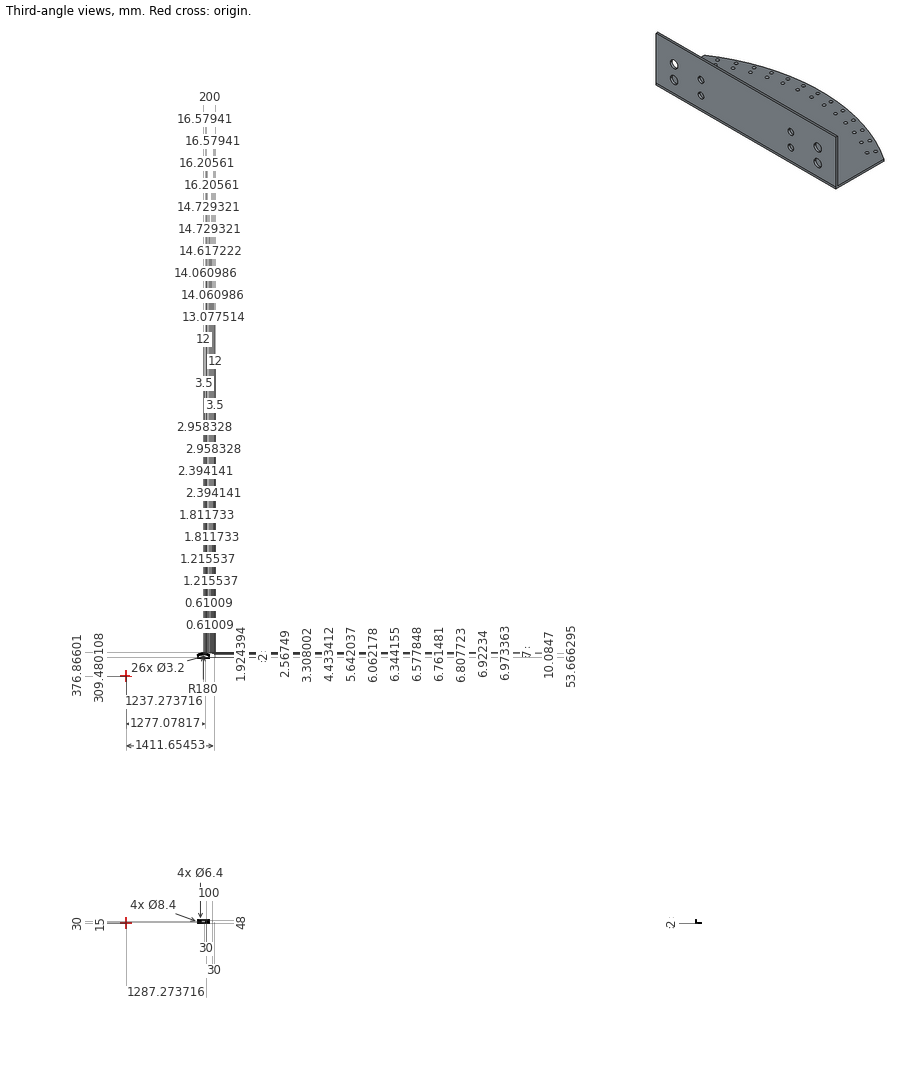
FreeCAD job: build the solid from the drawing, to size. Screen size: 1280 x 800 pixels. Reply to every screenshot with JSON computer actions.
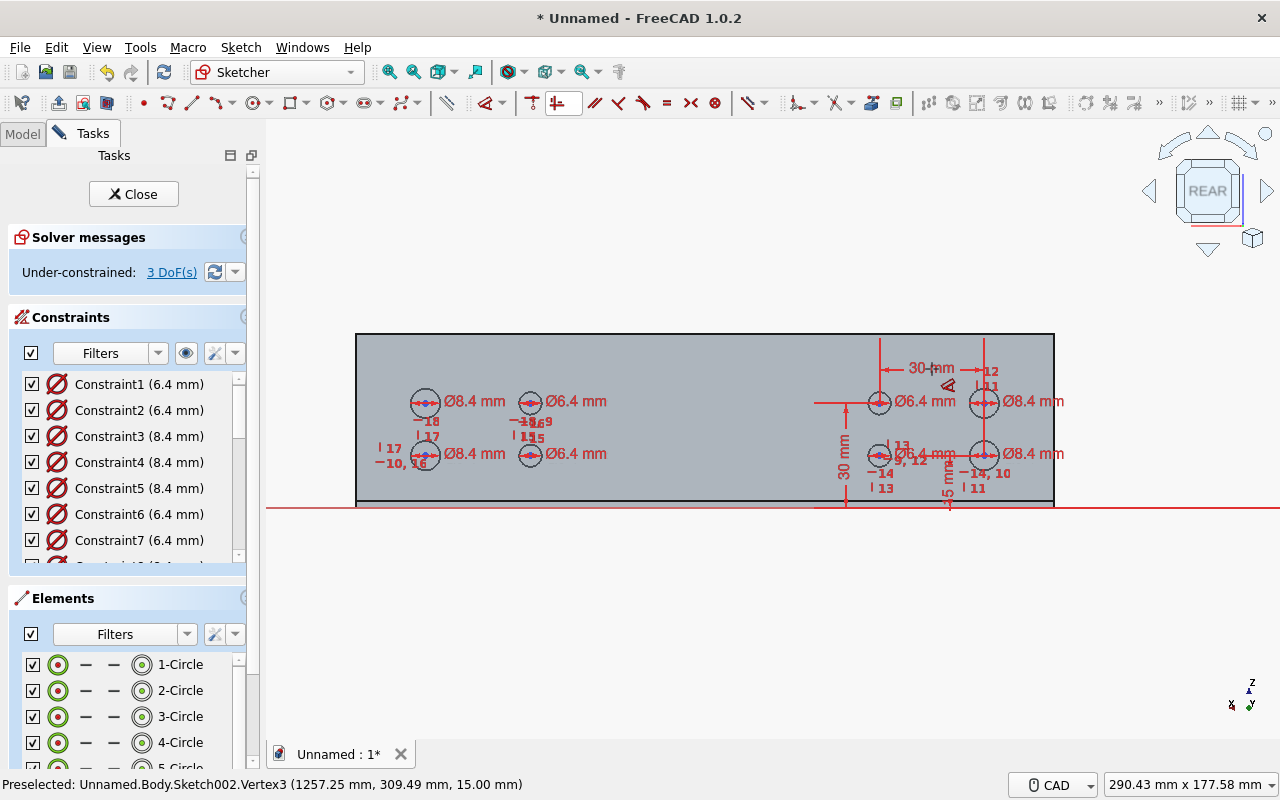
{"action": "left_click", "coordinate": [530, 403]}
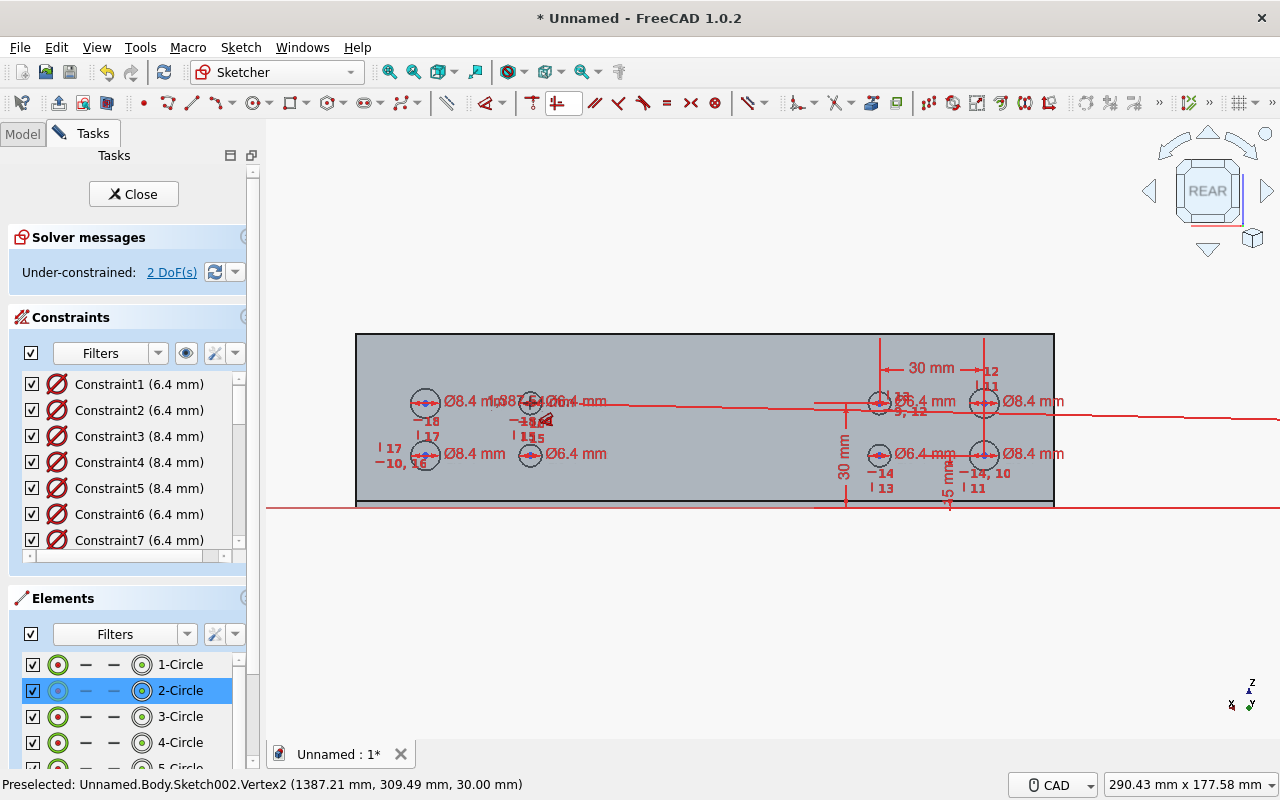
{"action": "left_click", "coordinate": [426, 456]}
{"action": "left_click", "coordinate": [478, 490]}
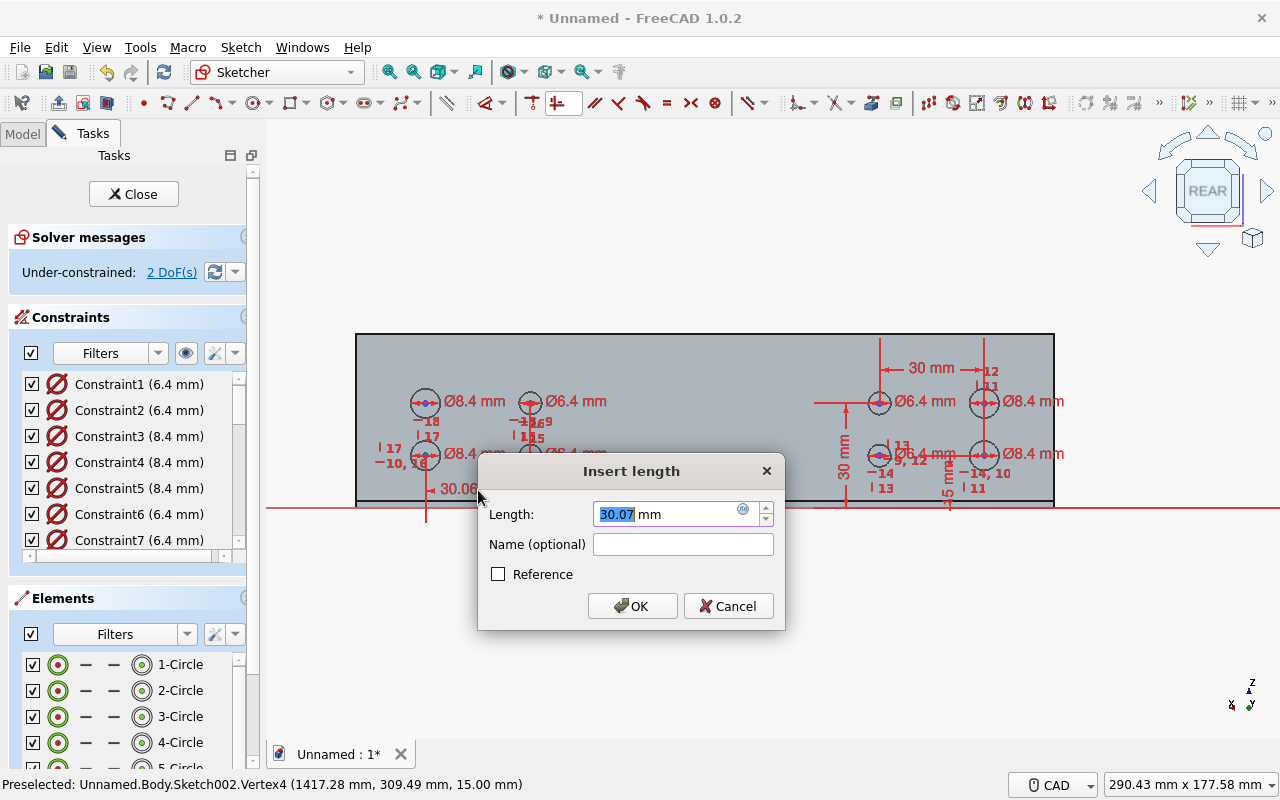
{"action": "type", "text": "30"}
{"action": "key", "text": "Return"}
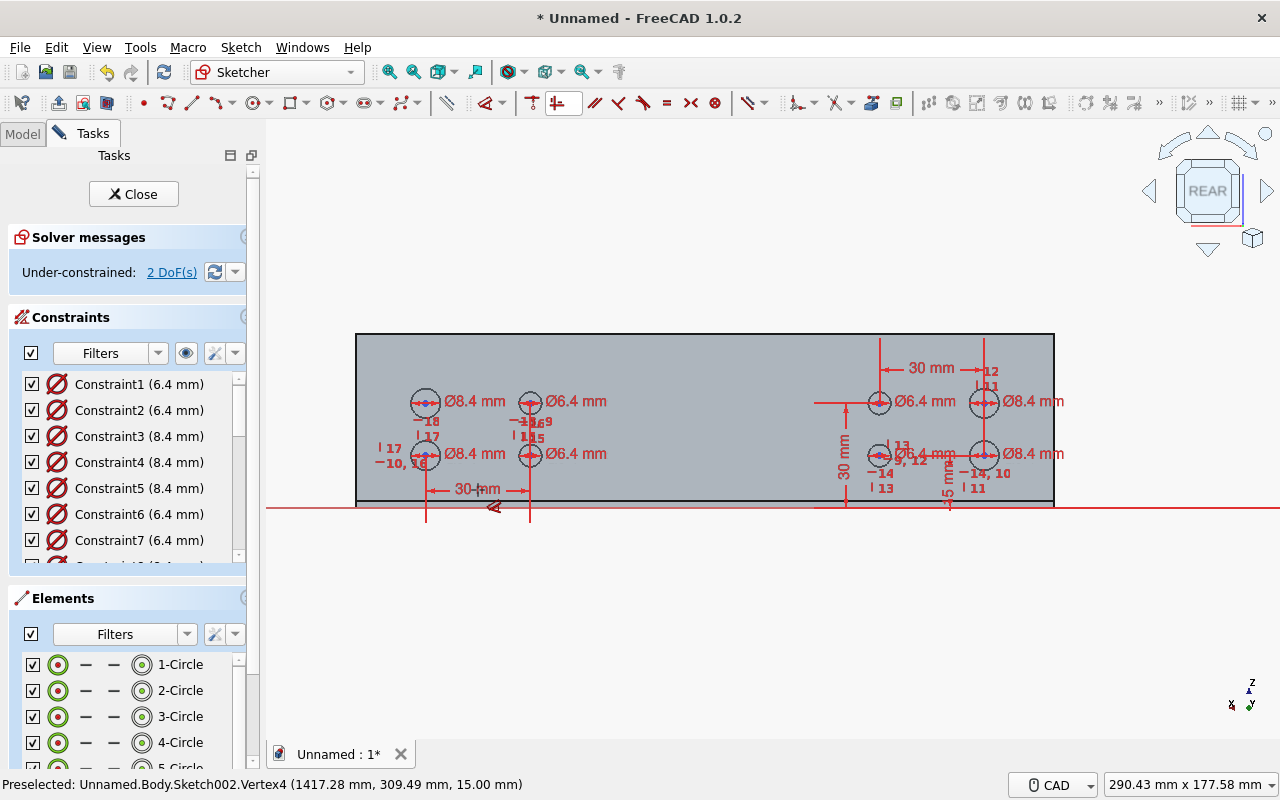
{"action": "left_click", "coordinate": [880, 403]}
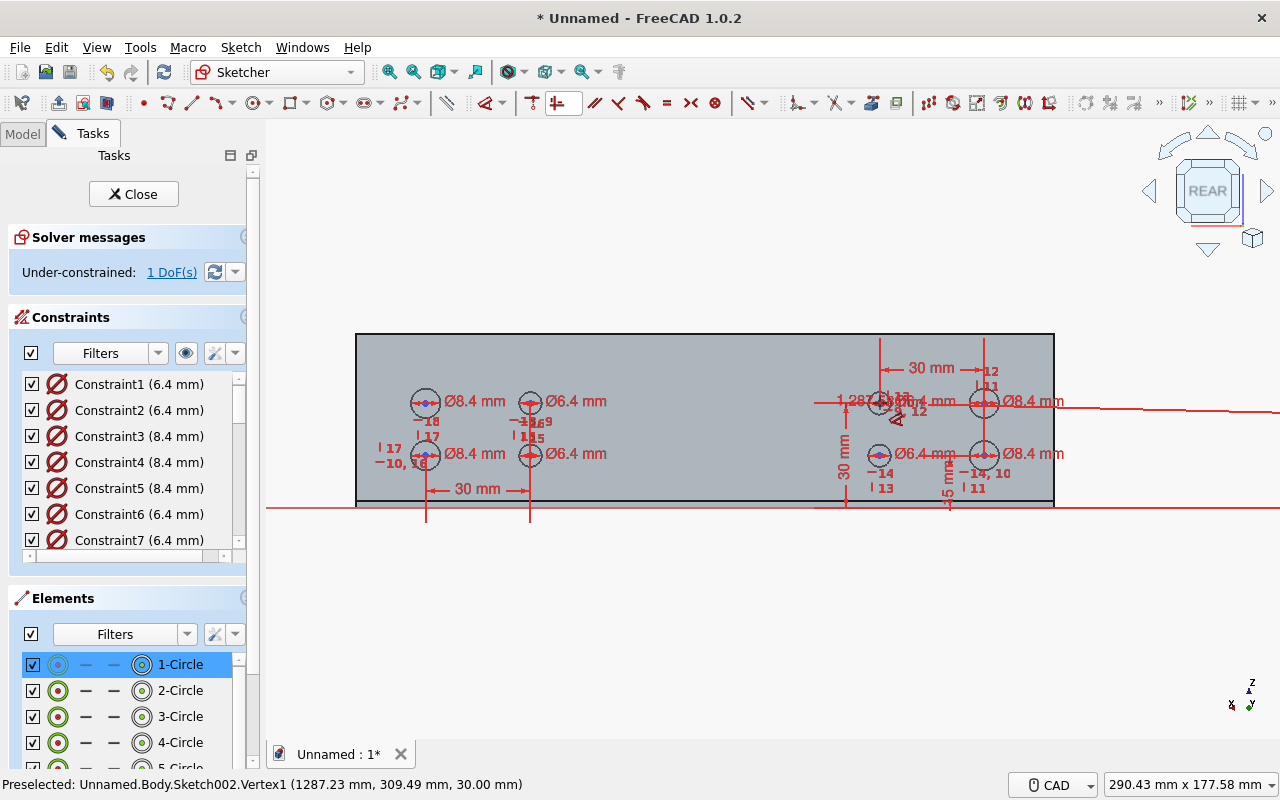
{"action": "left_click", "coordinate": [530, 403]}
{"action": "left_click", "coordinate": [705, 369]}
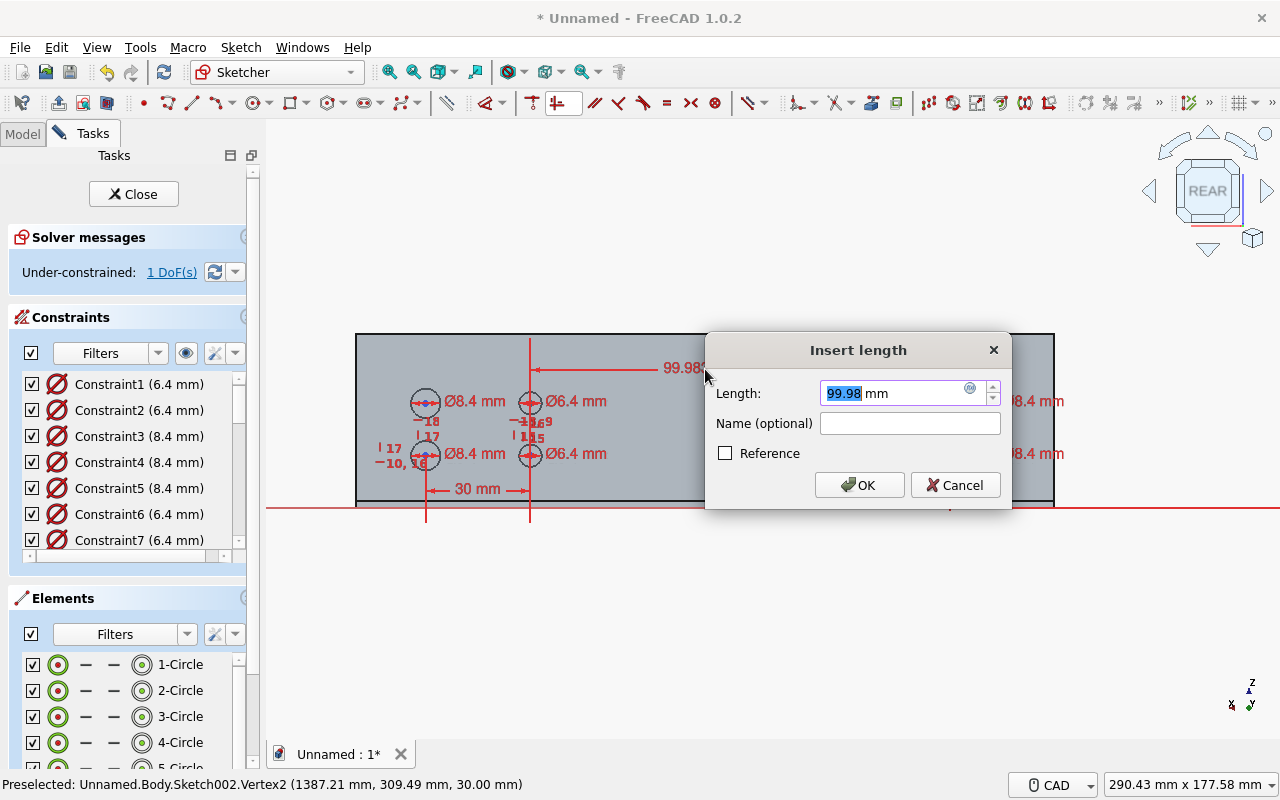
{"action": "type", "text": "100"}
{"action": "key", "text": "Return"}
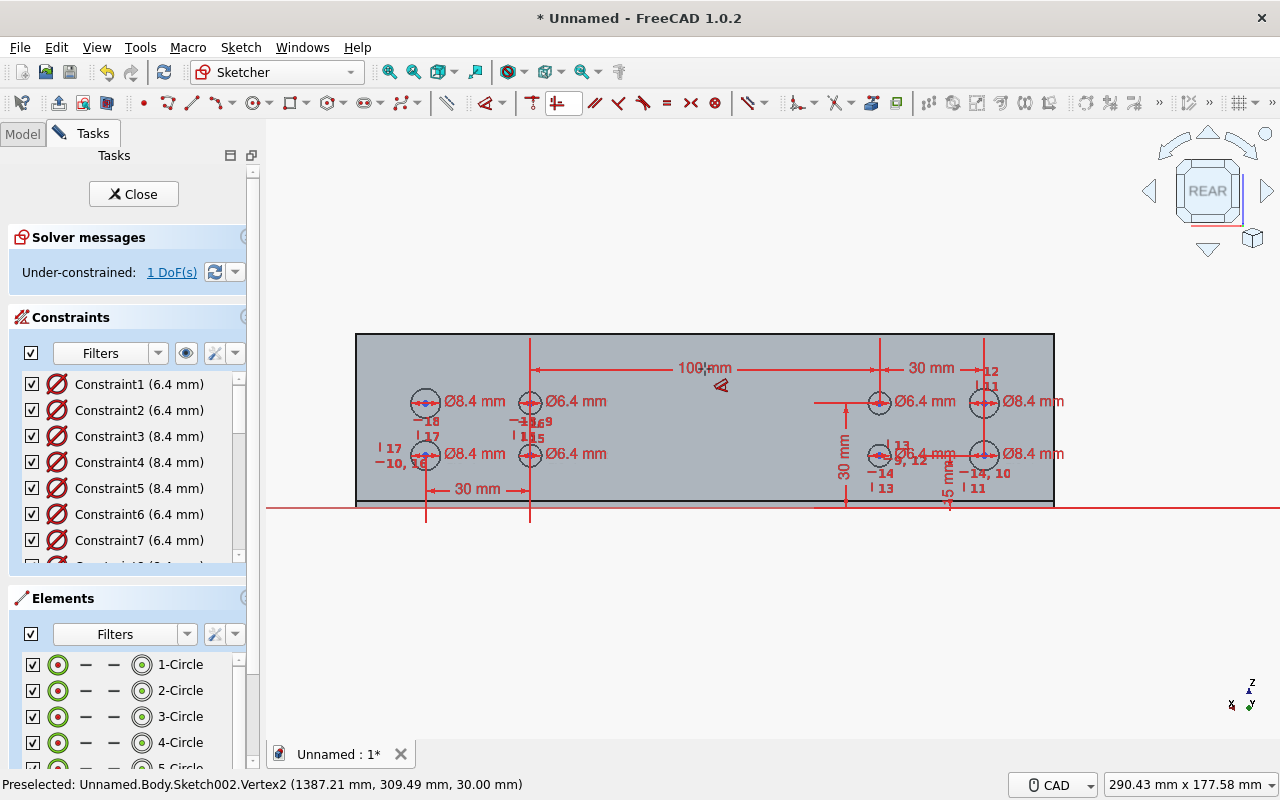
{"action": "left_click", "coordinate": [880, 403]}
{"action": "left_click", "coordinate": [997, 542]}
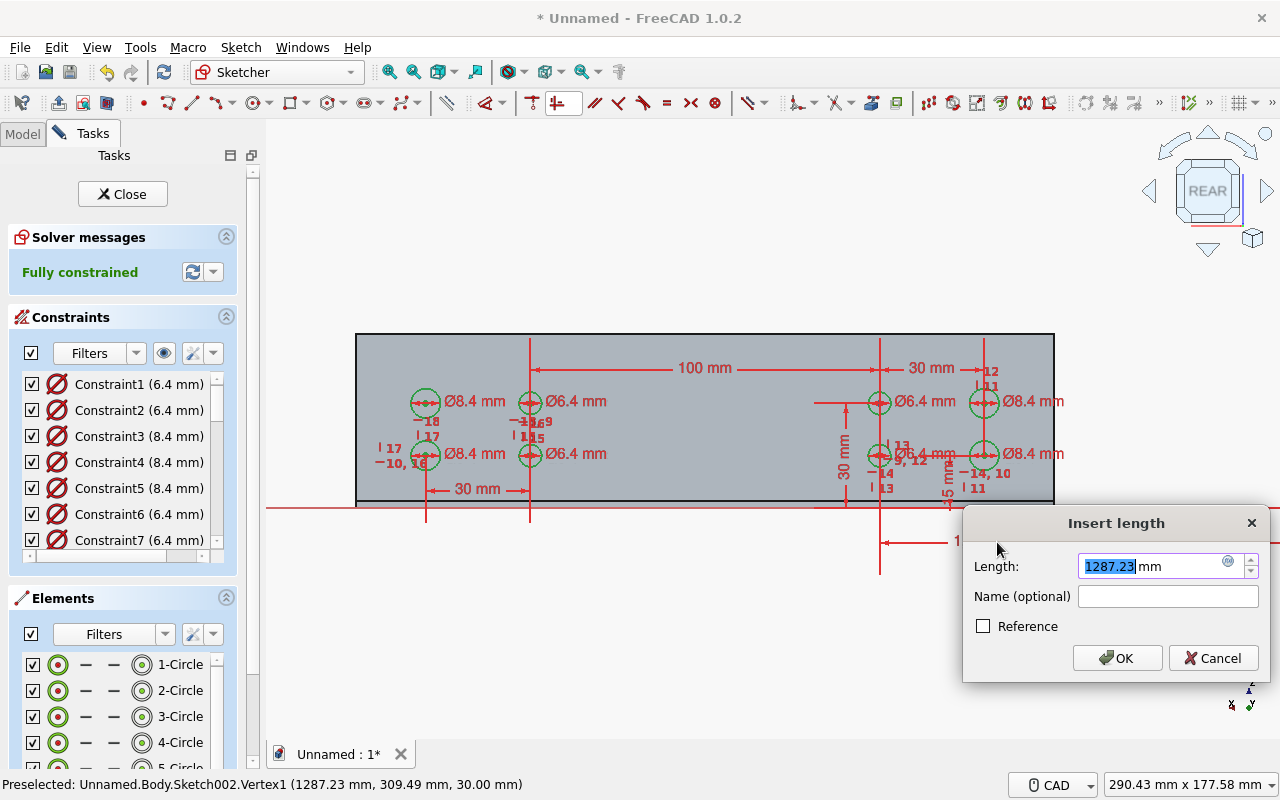
{"action": "type", "text": "1287.273716"}
{"action": "key", "text": "Return"}
{"action": "key", "text": "Escape"}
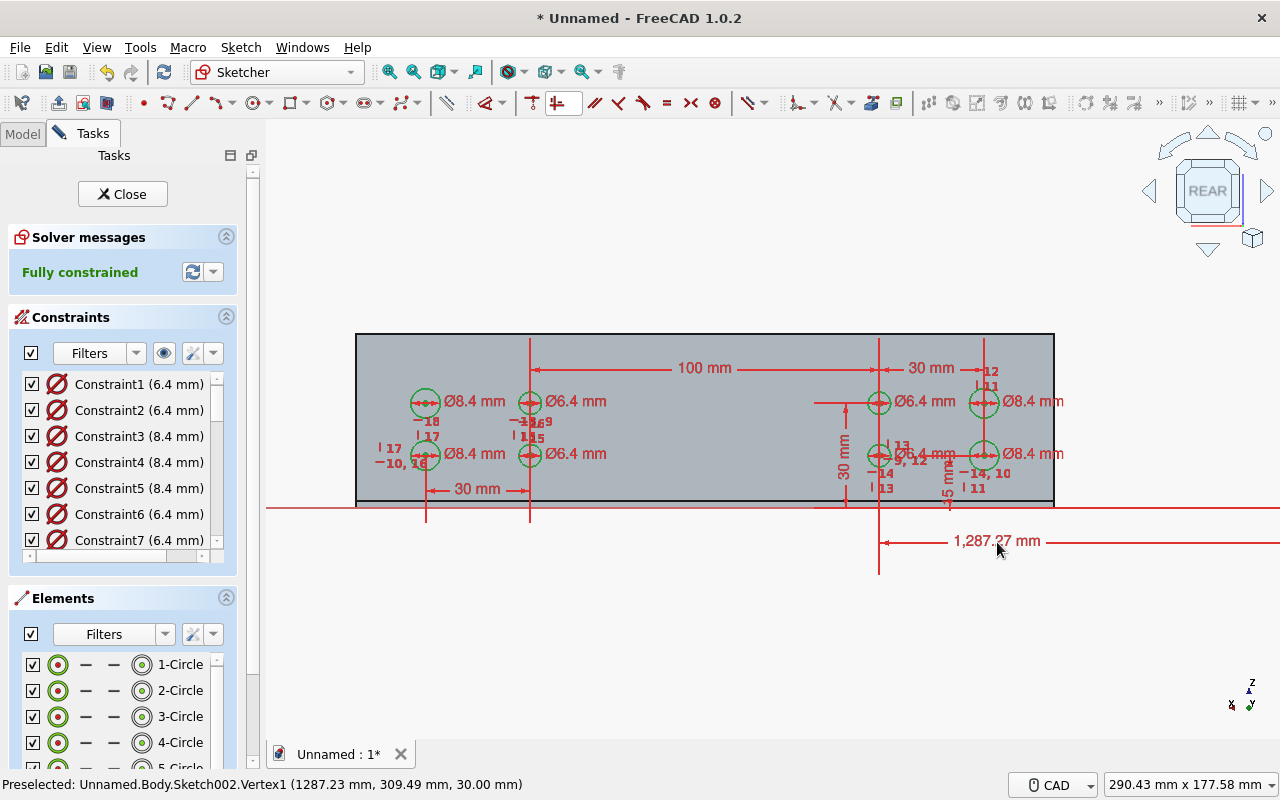
{"action": "left_click", "coordinate": [123, 194]}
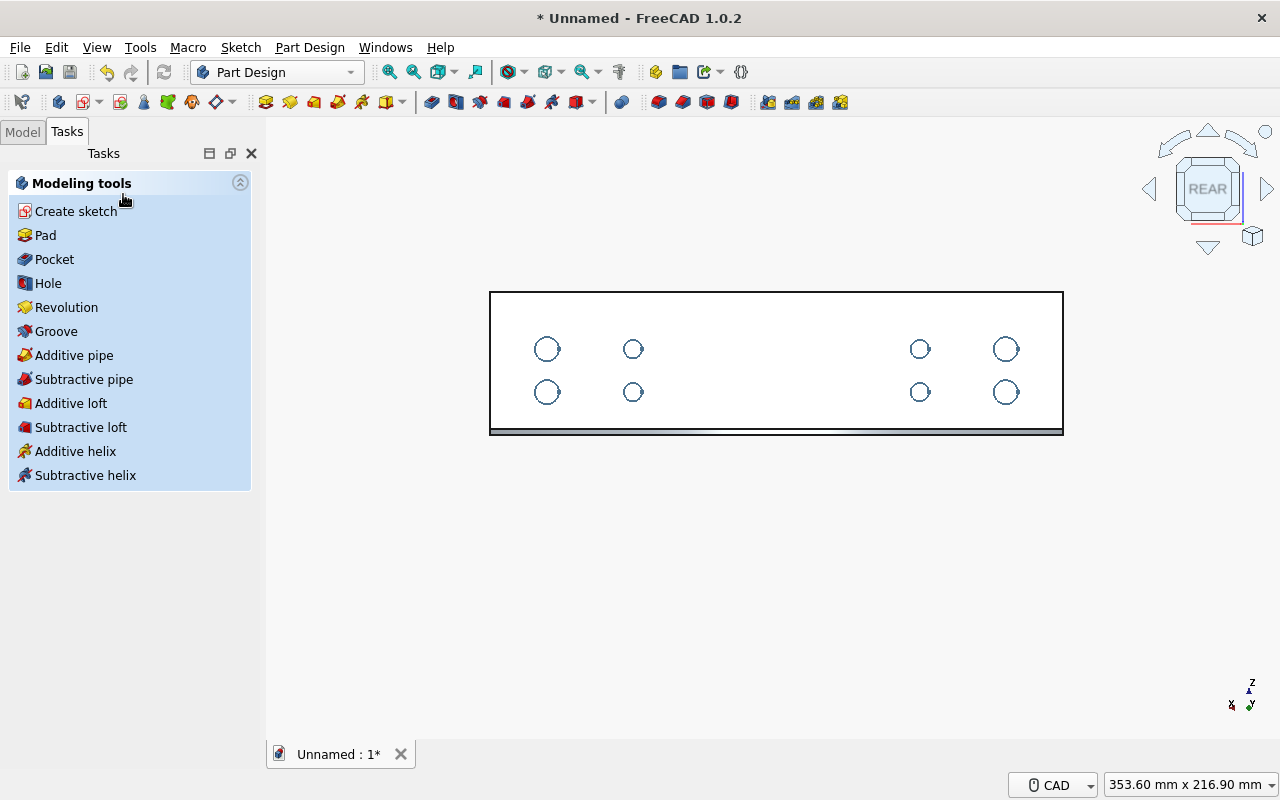
{"action": "left_click", "coordinate": [432, 102]}